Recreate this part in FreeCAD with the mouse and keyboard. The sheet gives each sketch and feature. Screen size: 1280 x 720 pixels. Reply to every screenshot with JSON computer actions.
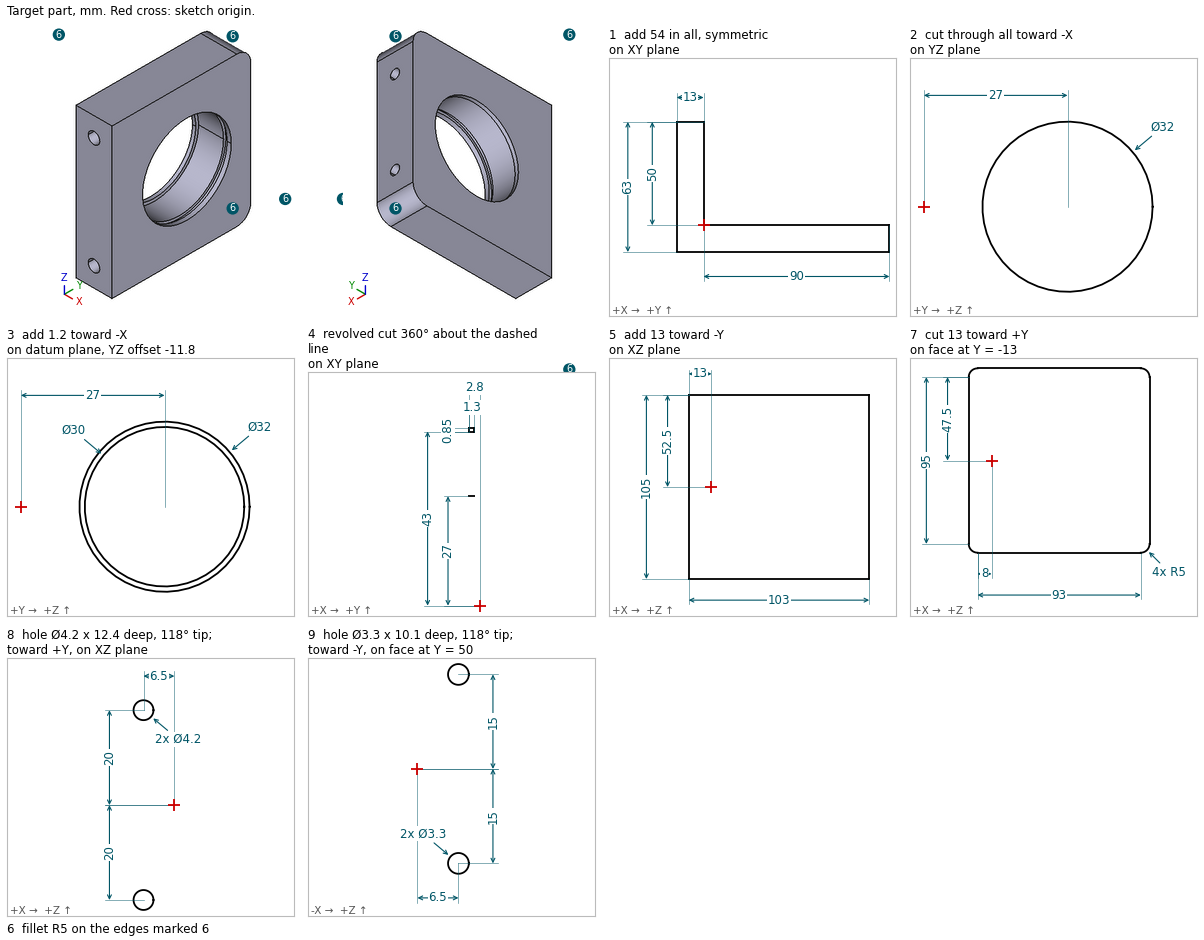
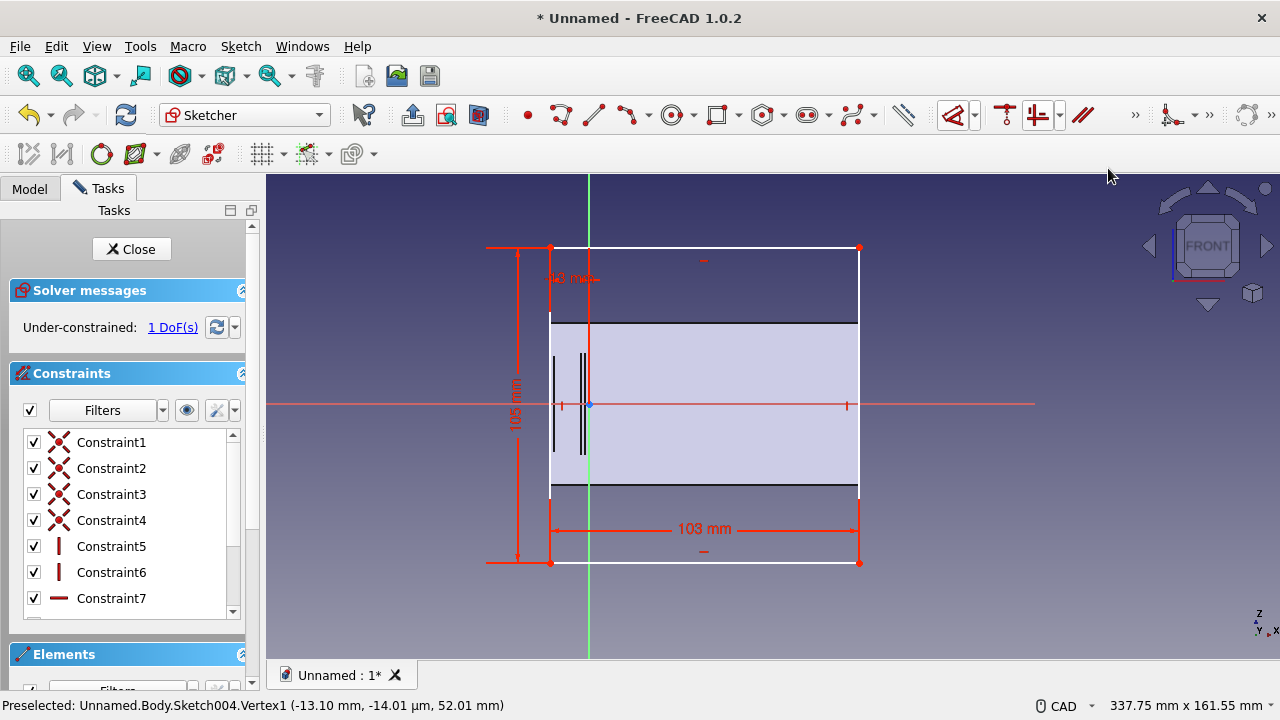
{"action": "left_click", "coordinate": [550, 248]}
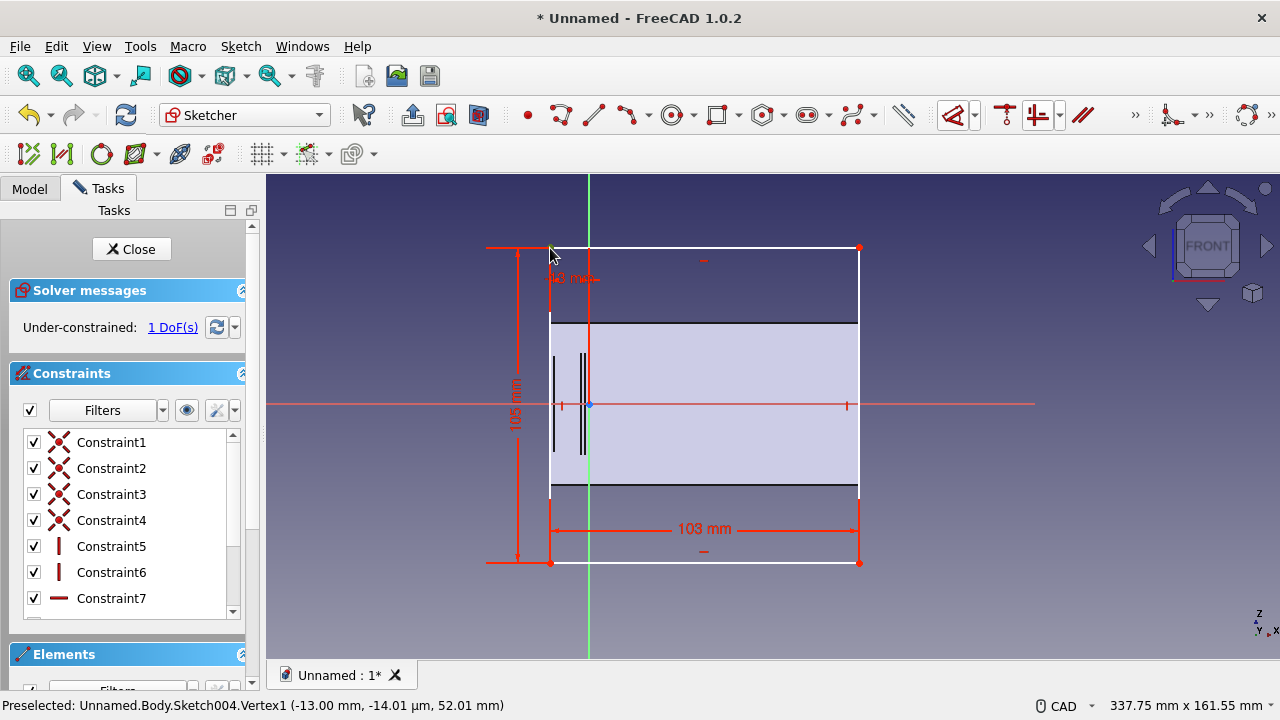
{"action": "left_click", "coordinate": [974, 116]}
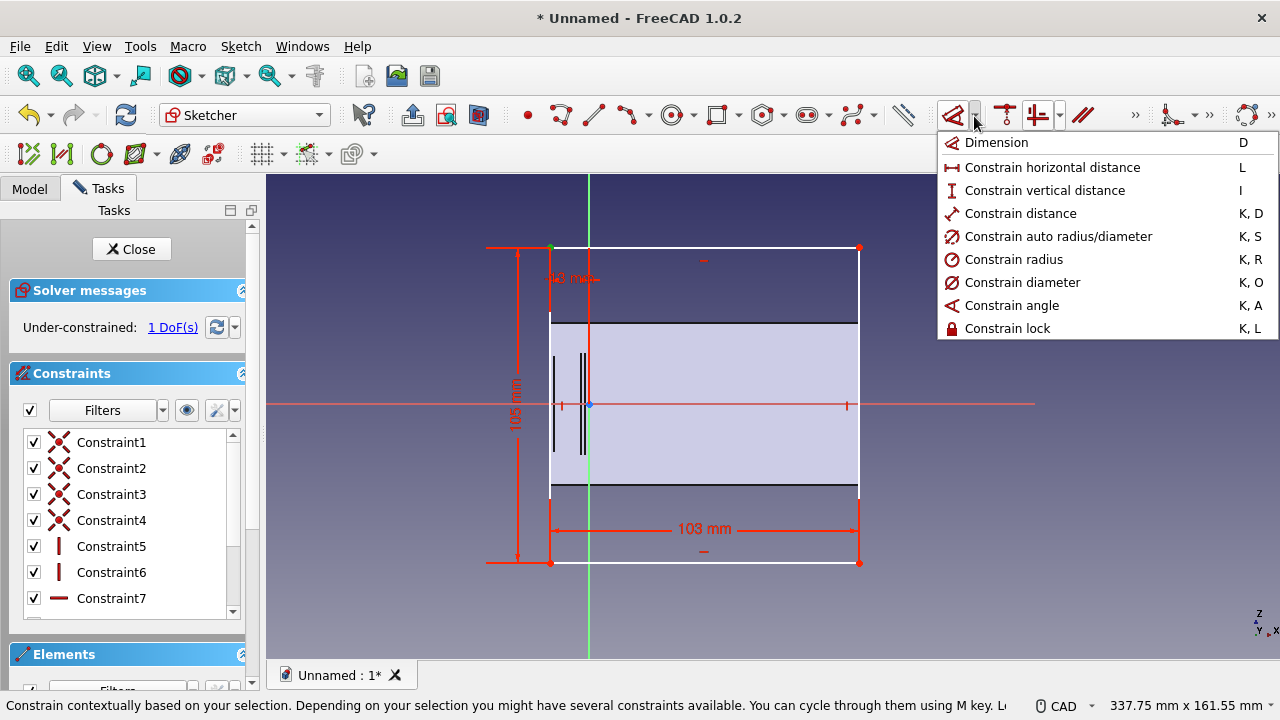
{"action": "left_click", "coordinate": [1108, 190]}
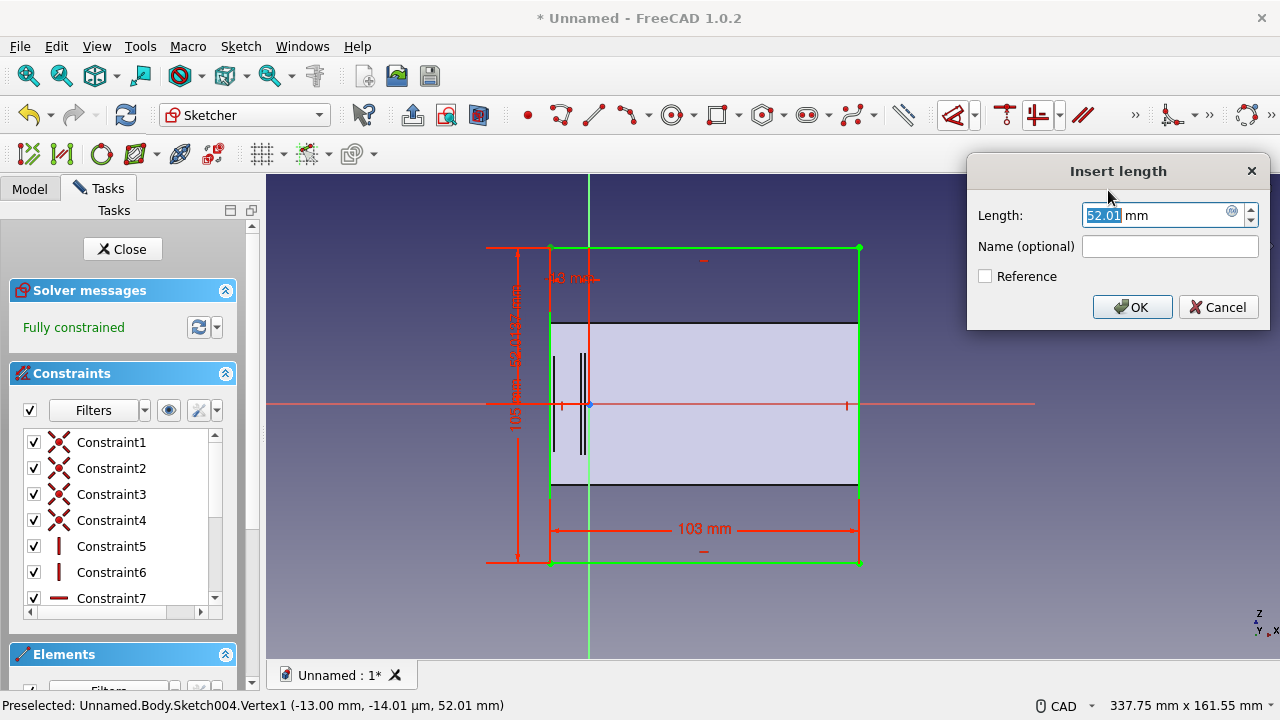
{"action": "type", "text": "52.5"}
{"action": "key", "text": "Return"}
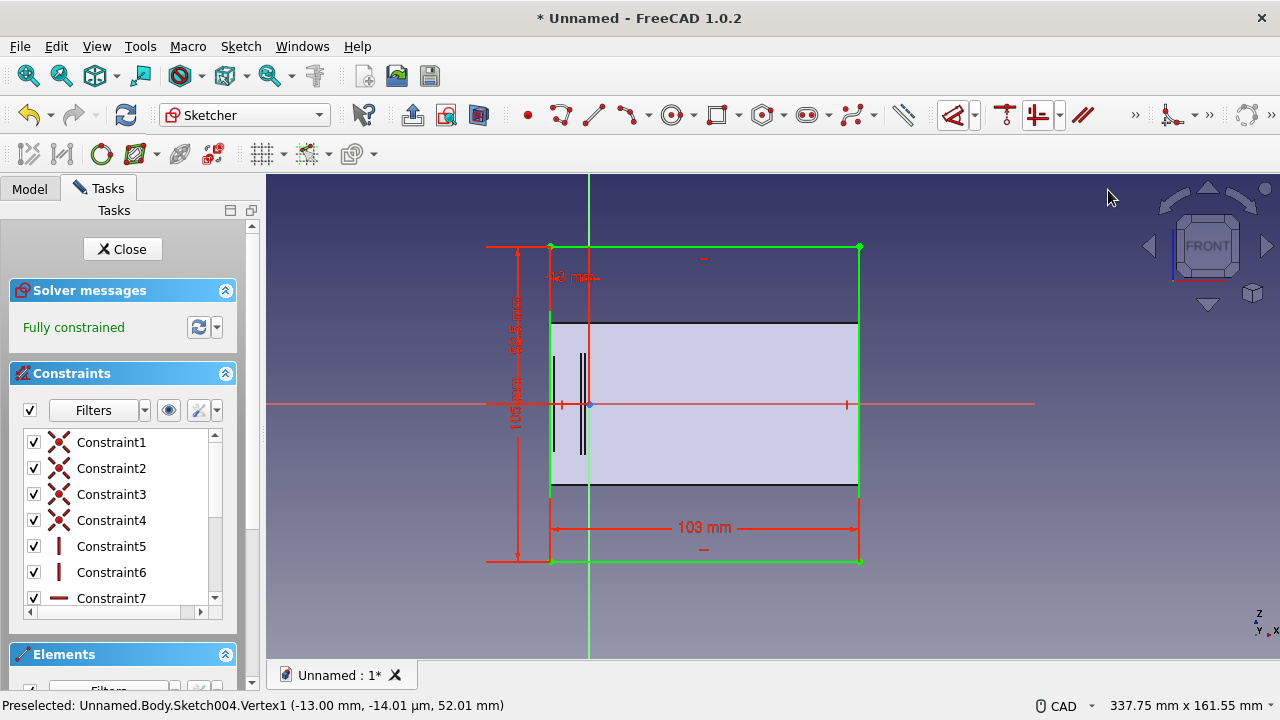
{"action": "left_click", "coordinate": [123, 249]}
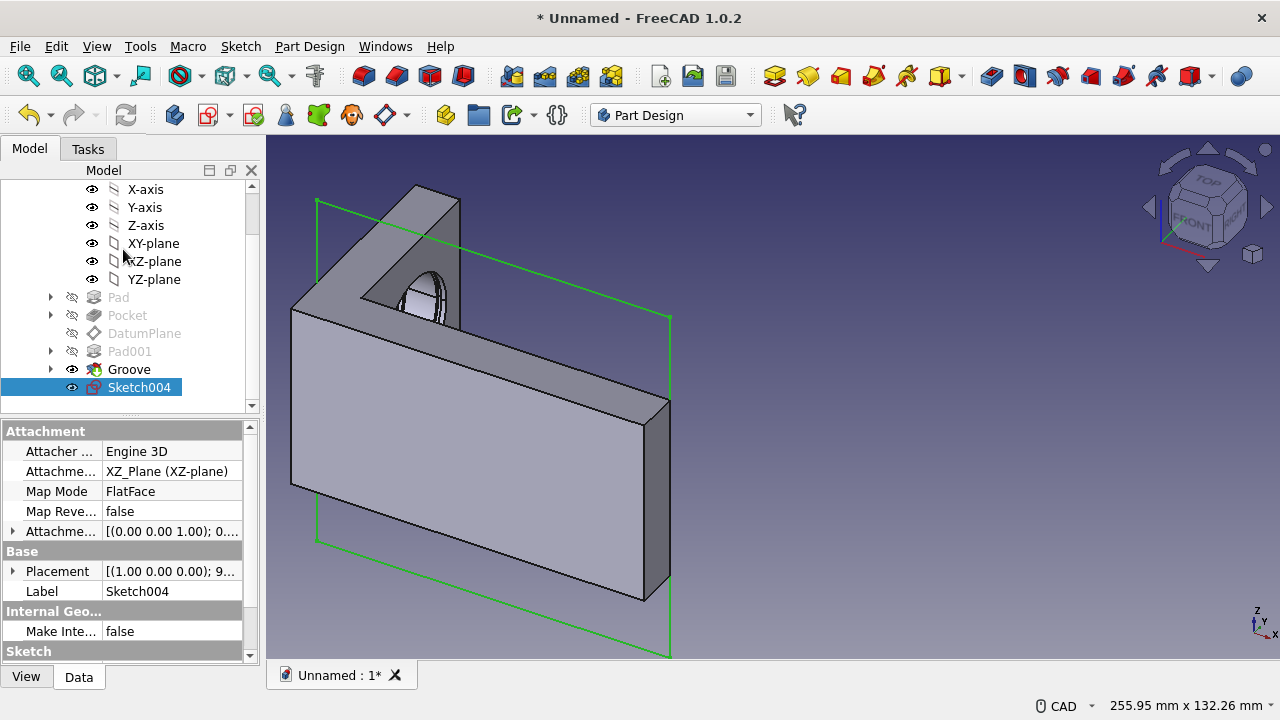
{"action": "left_click", "coordinate": [775, 76]}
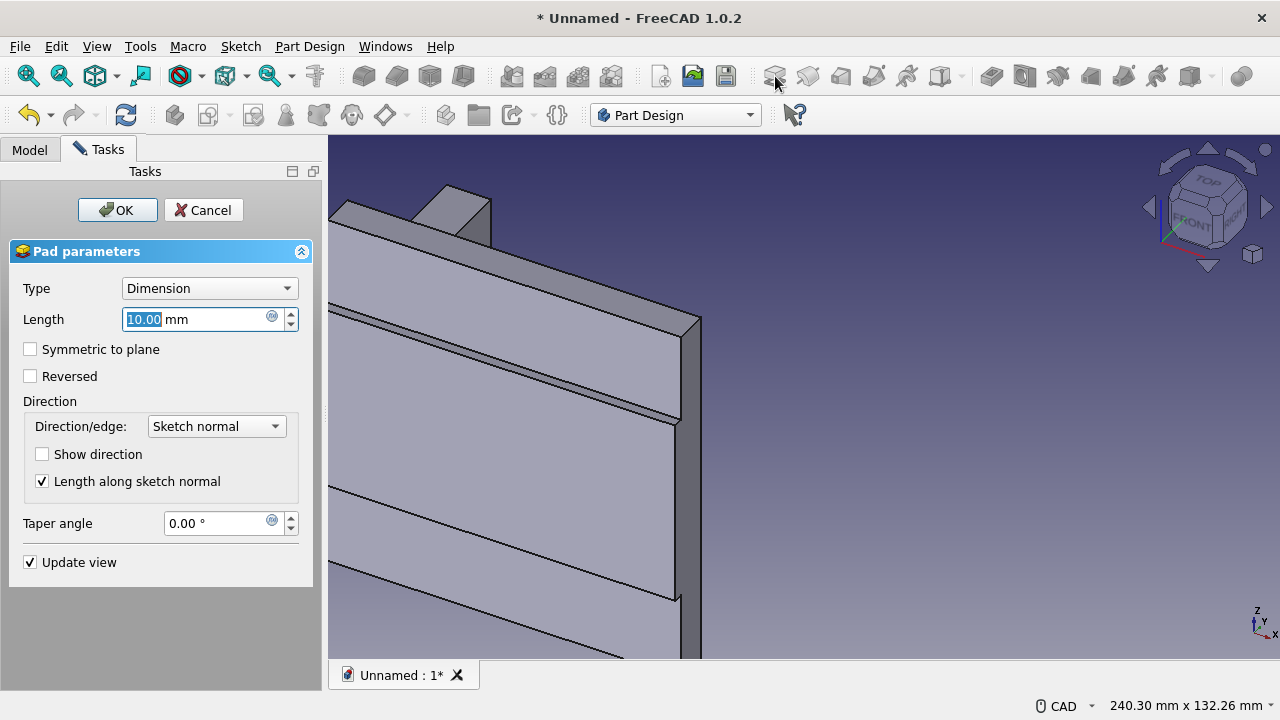
{"action": "type", "text": "13"}
{"action": "key", "text": "Tab"}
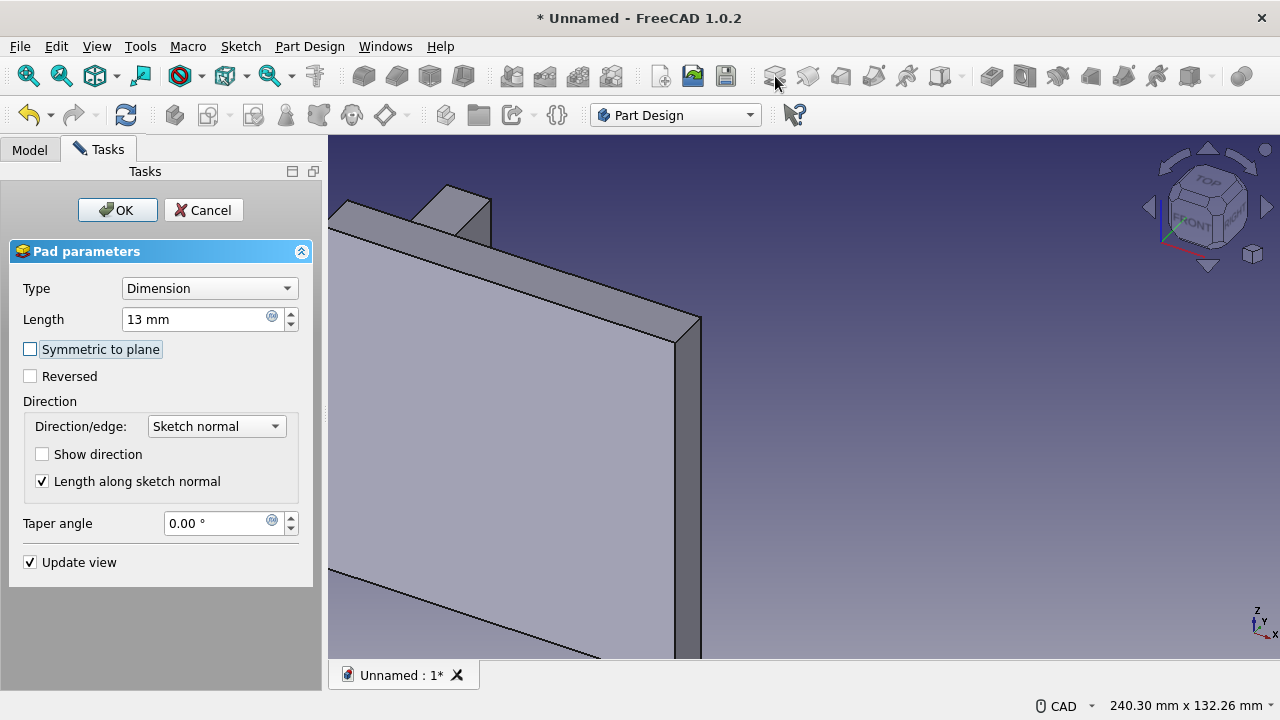
{"action": "left_click", "coordinate": [118, 210]}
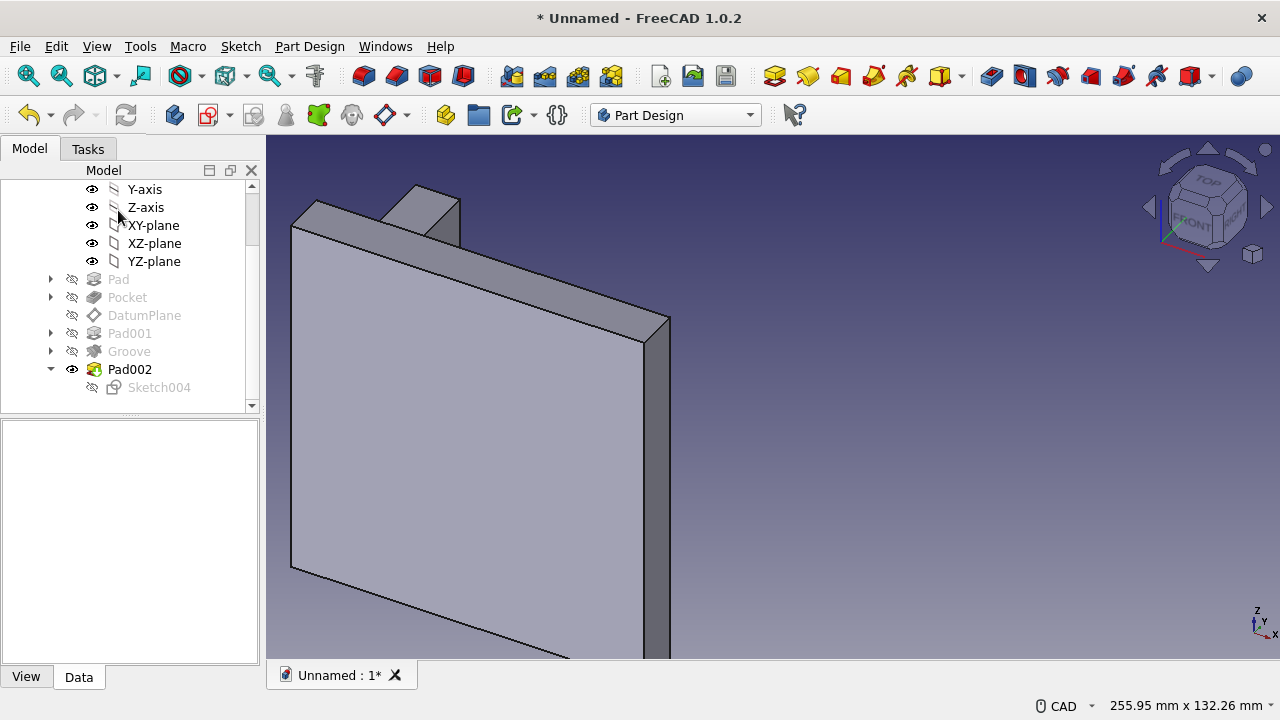
{"action": "left_click", "coordinate": [29, 76]}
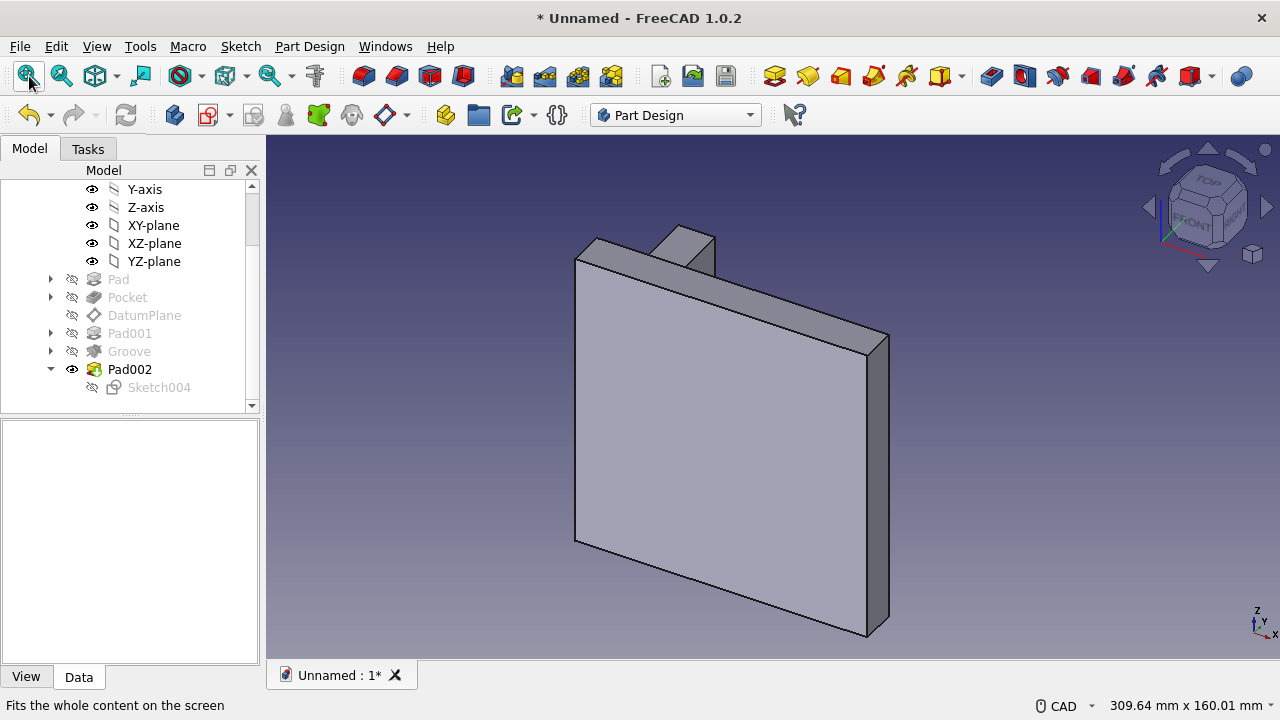
{"action": "left_click", "coordinate": [878, 344]}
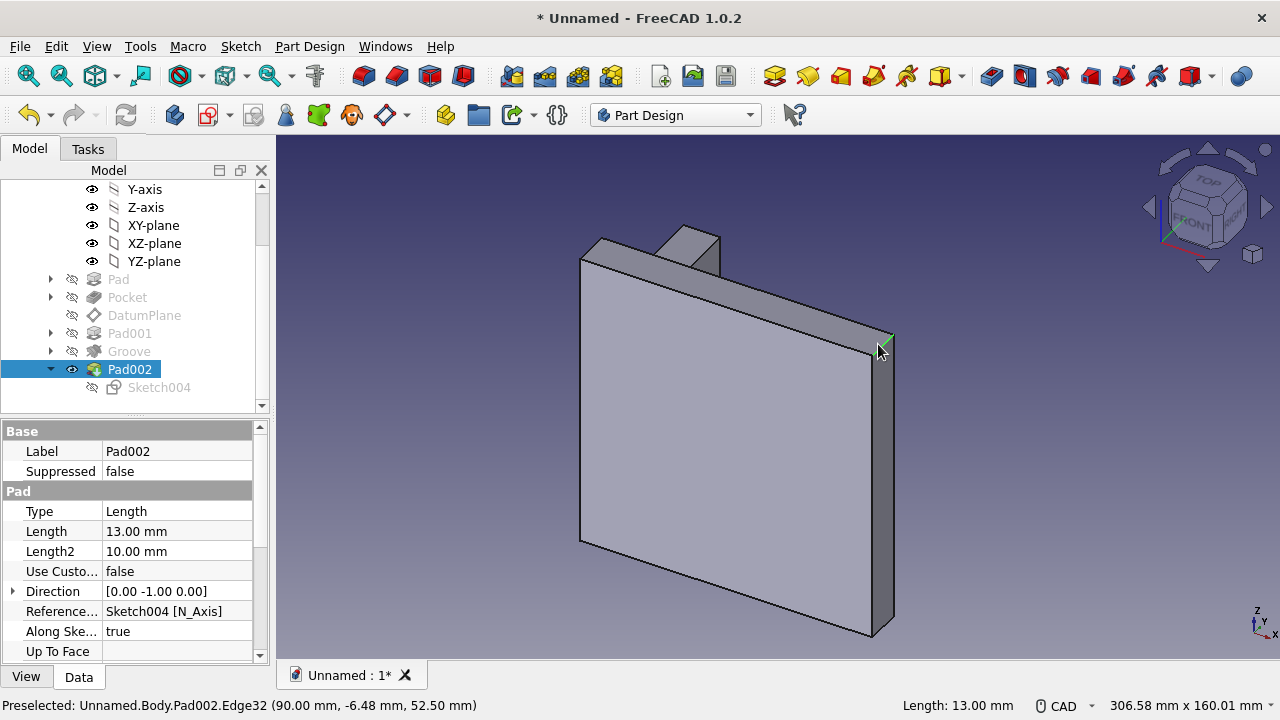
{"action": "key", "text": "0"}